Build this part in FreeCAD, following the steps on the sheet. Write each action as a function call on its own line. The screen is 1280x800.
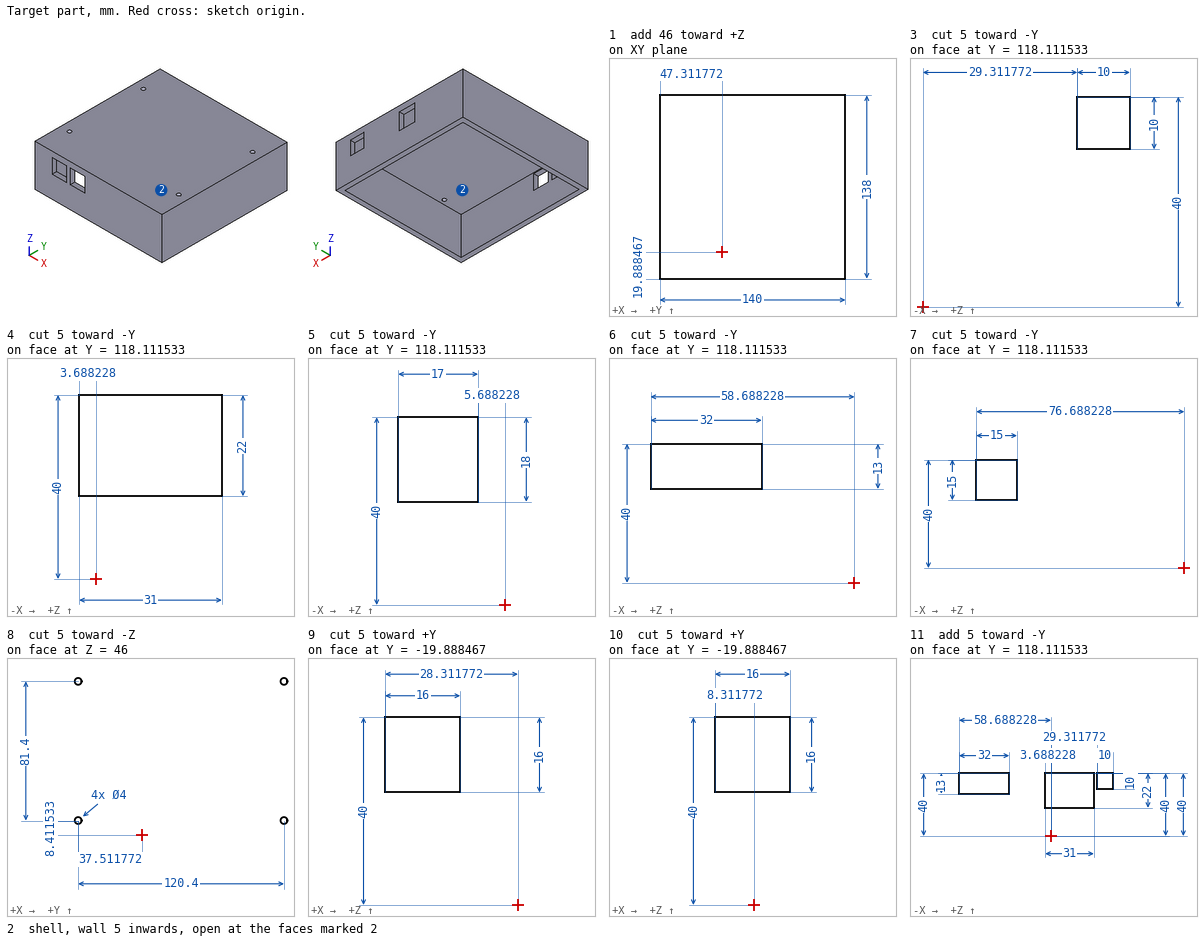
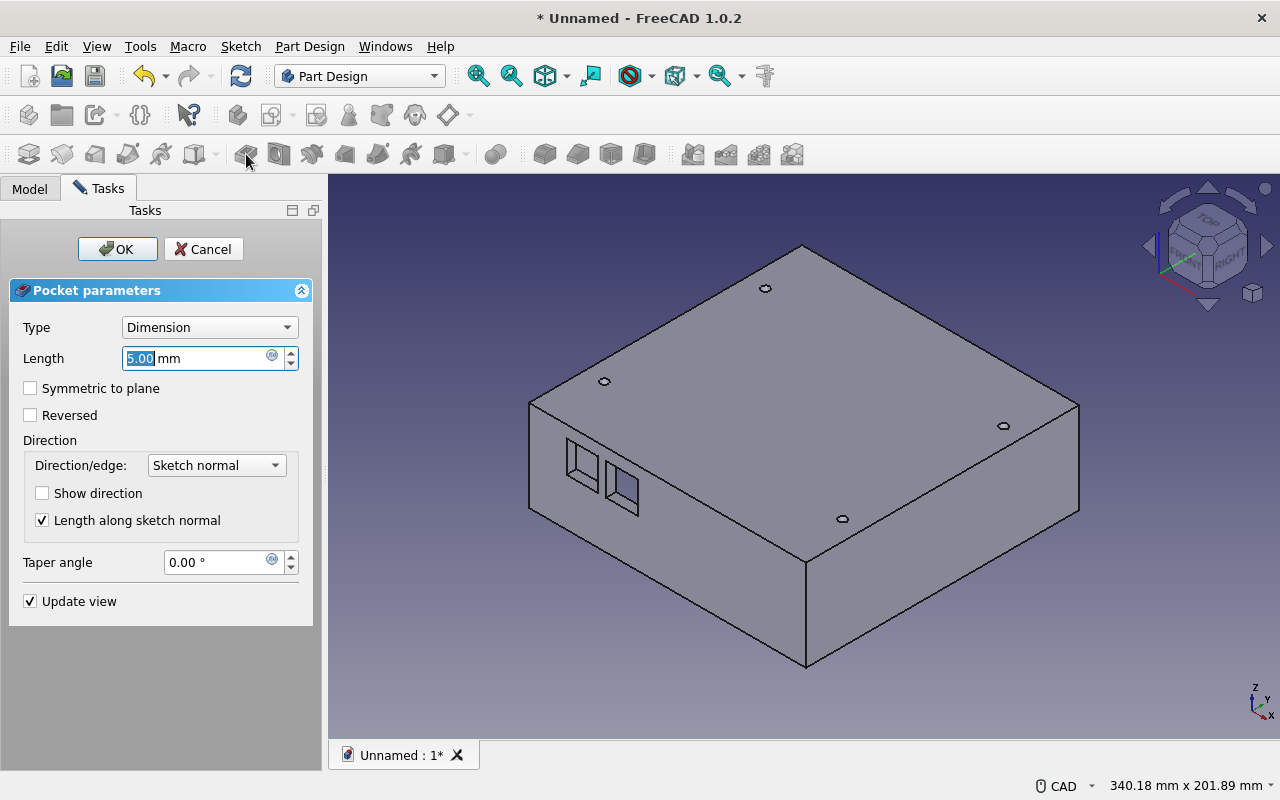
text(5)
key(Tab)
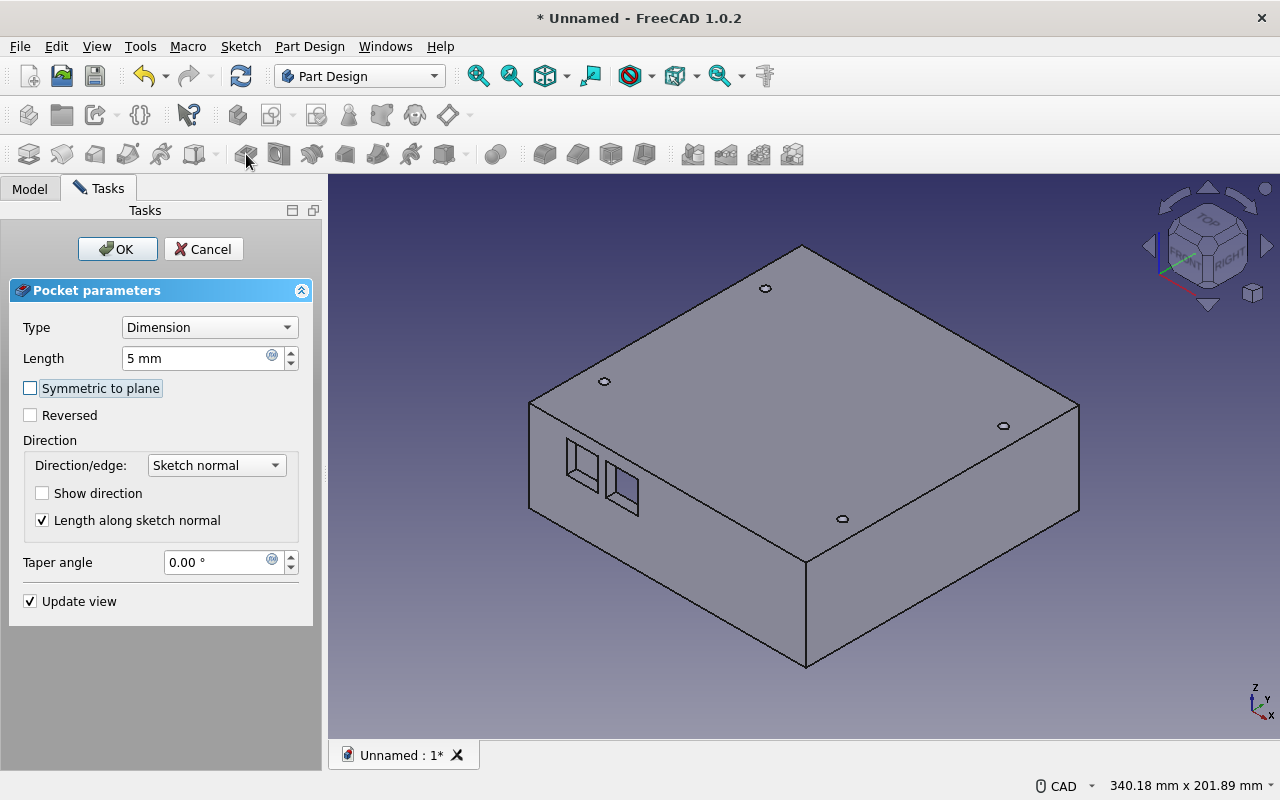
click(118, 249)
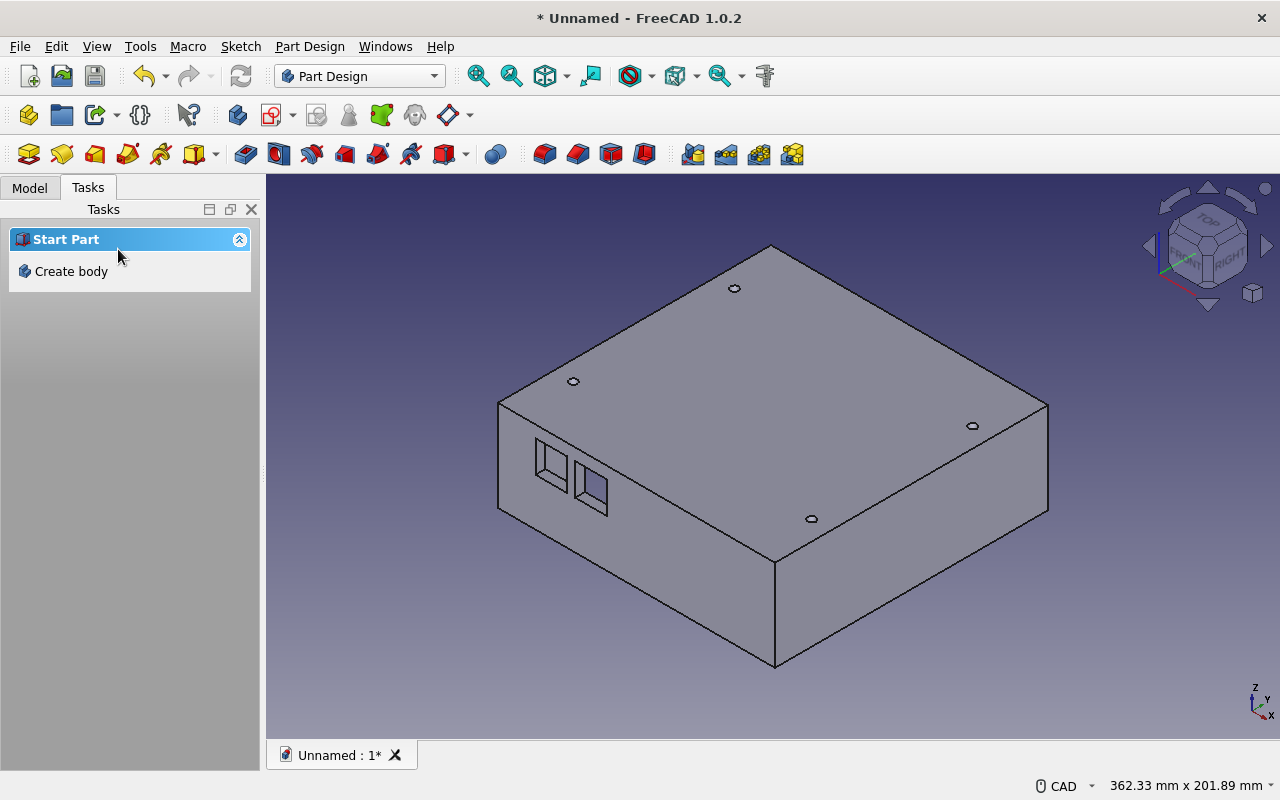
key(4)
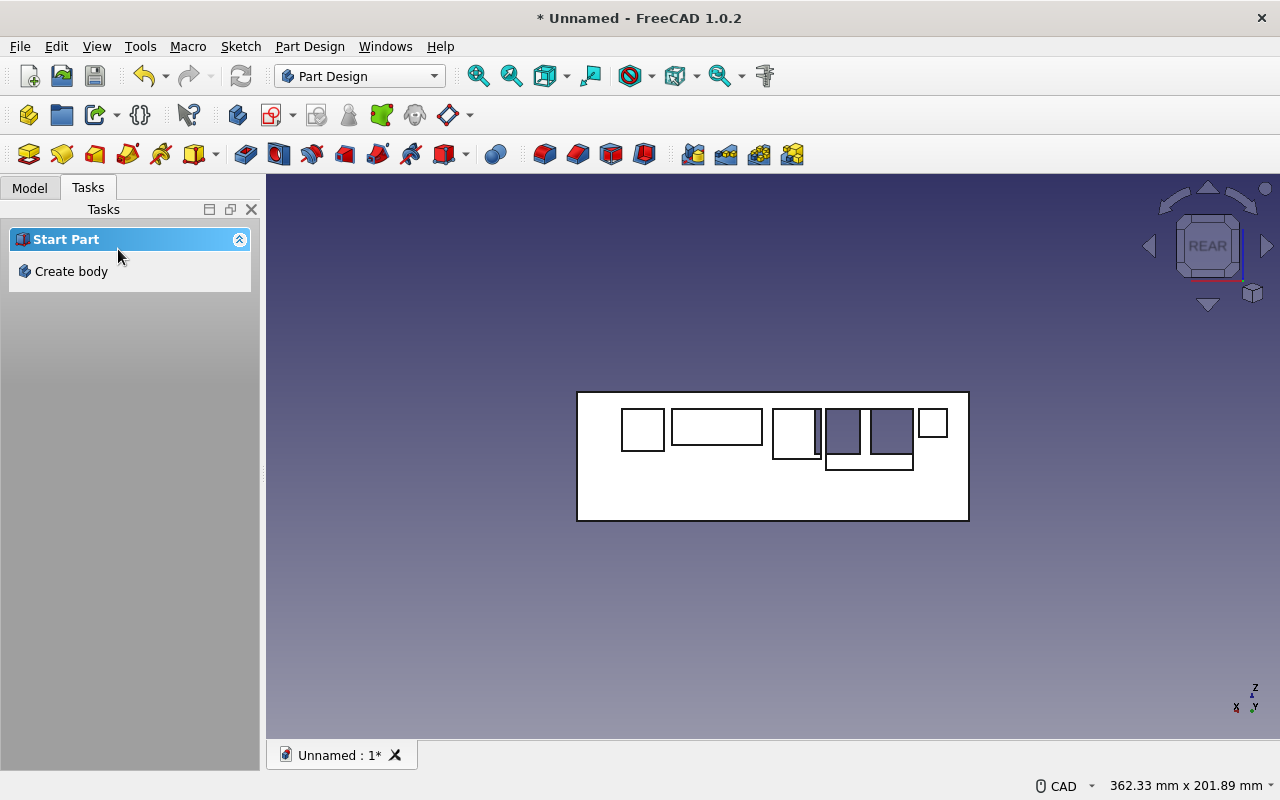
key(v)
key(f)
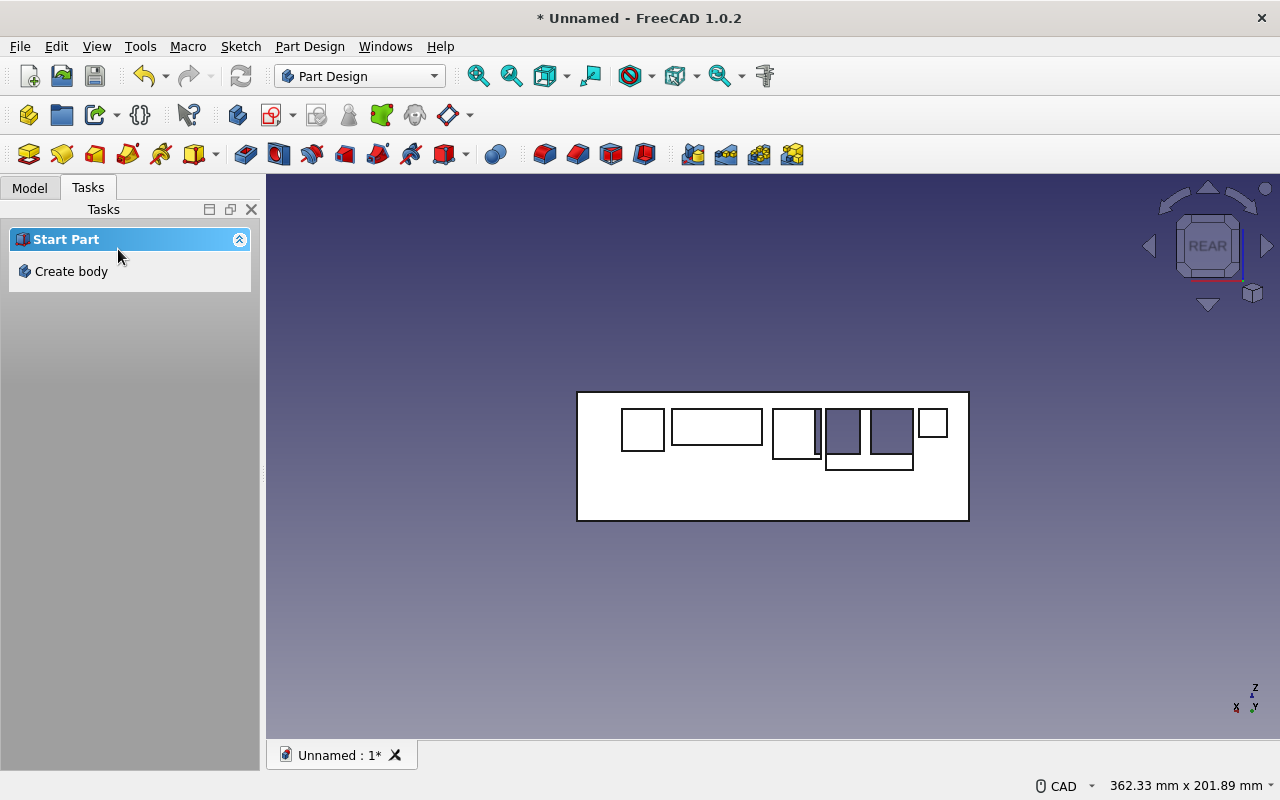
click(717, 474)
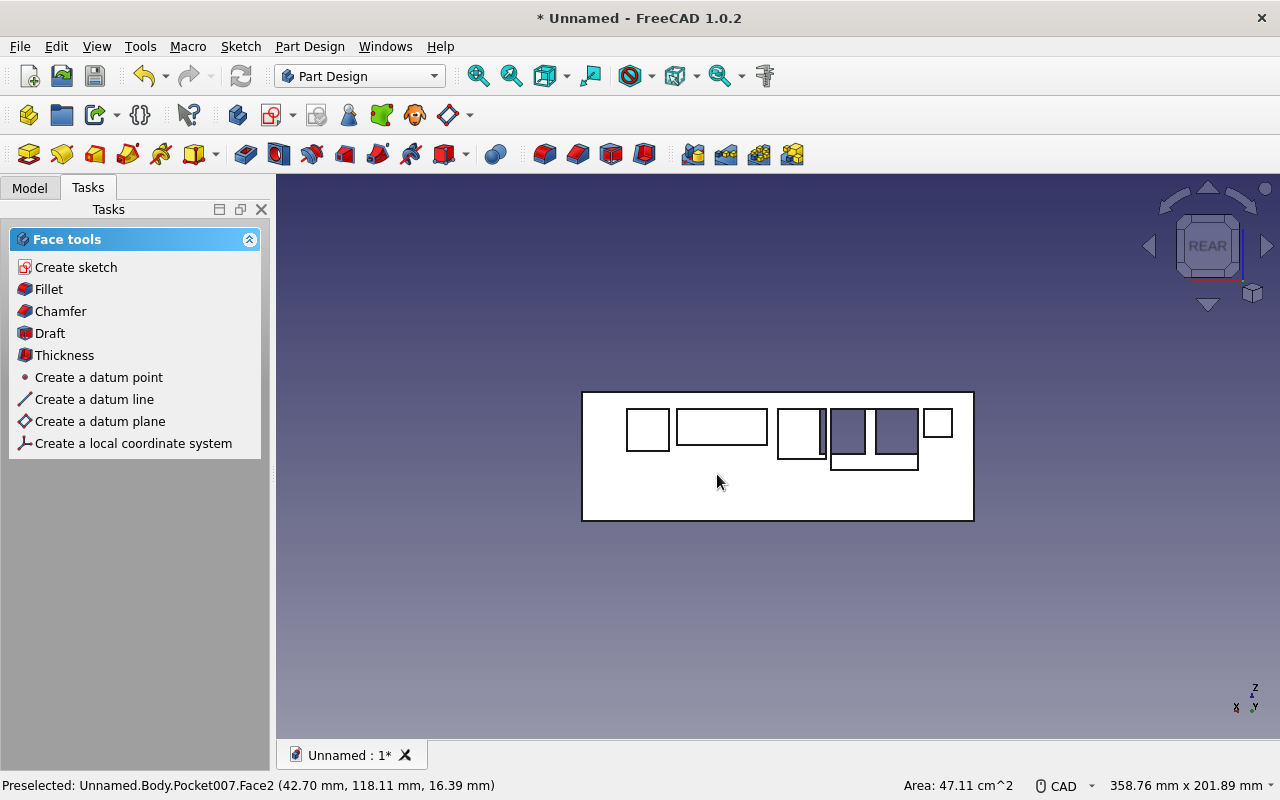
click(270, 116)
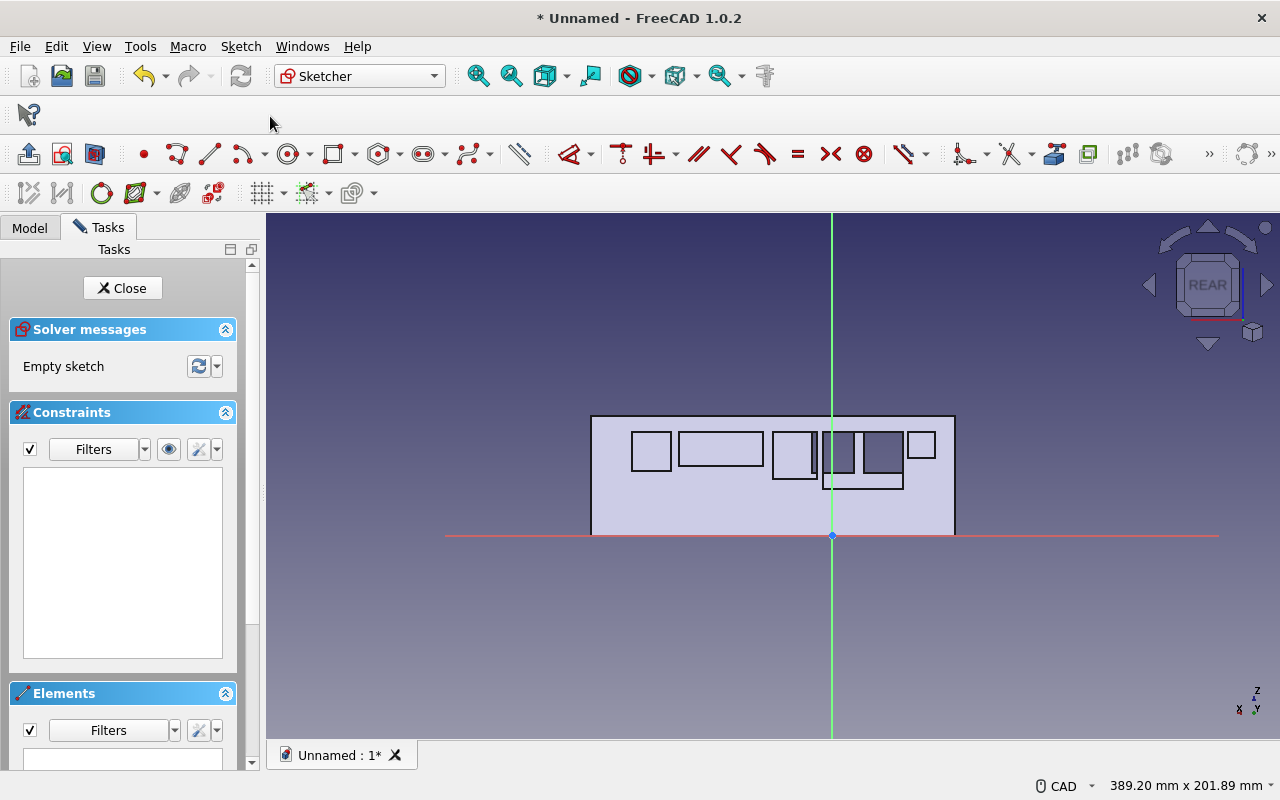
scroll(890, 490, up, 4)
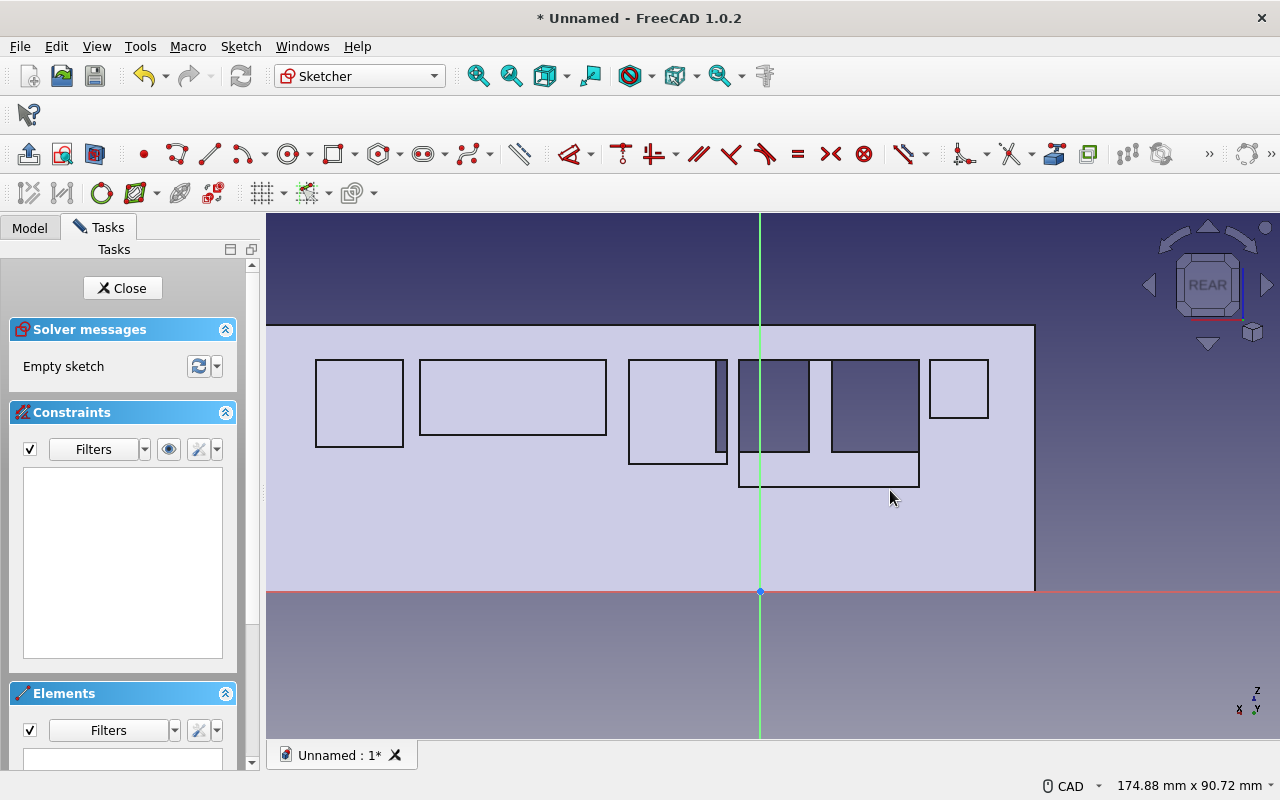
key(g)
key(r)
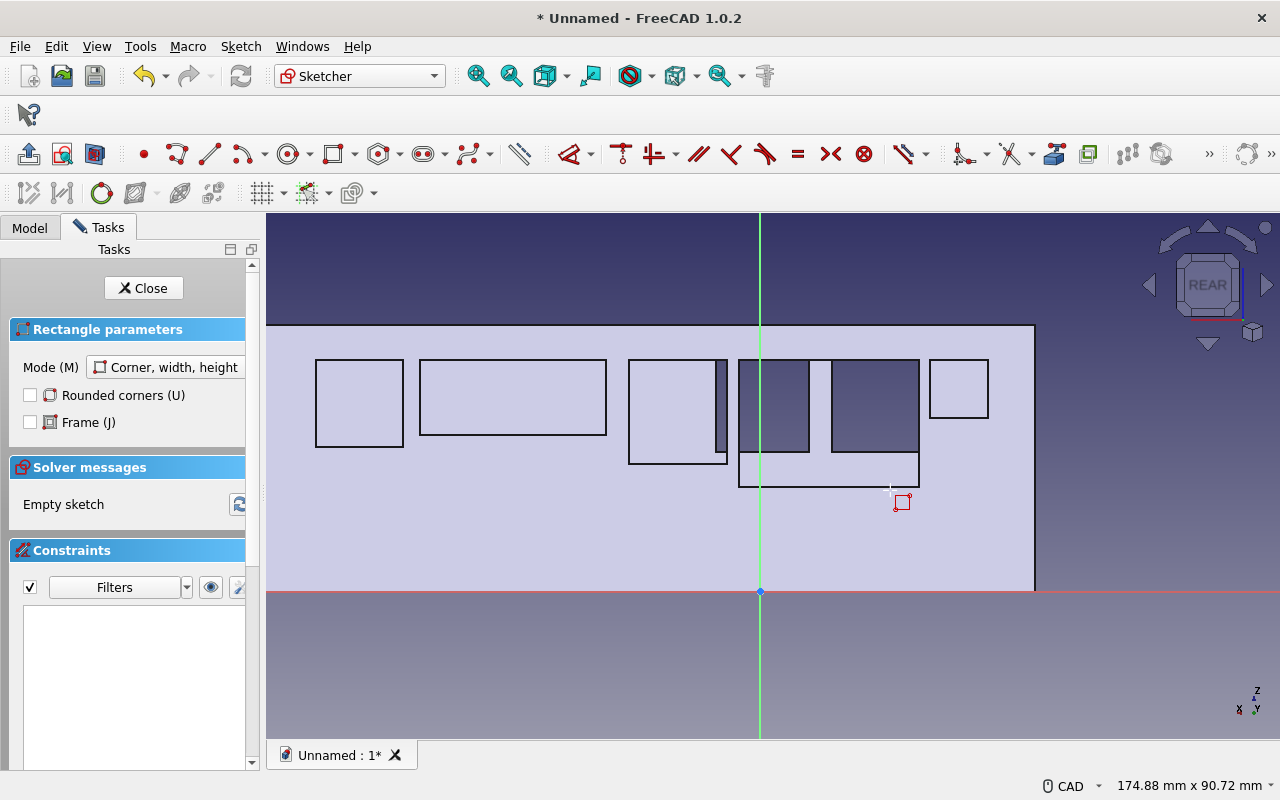
click(930, 360)
move(988, 418)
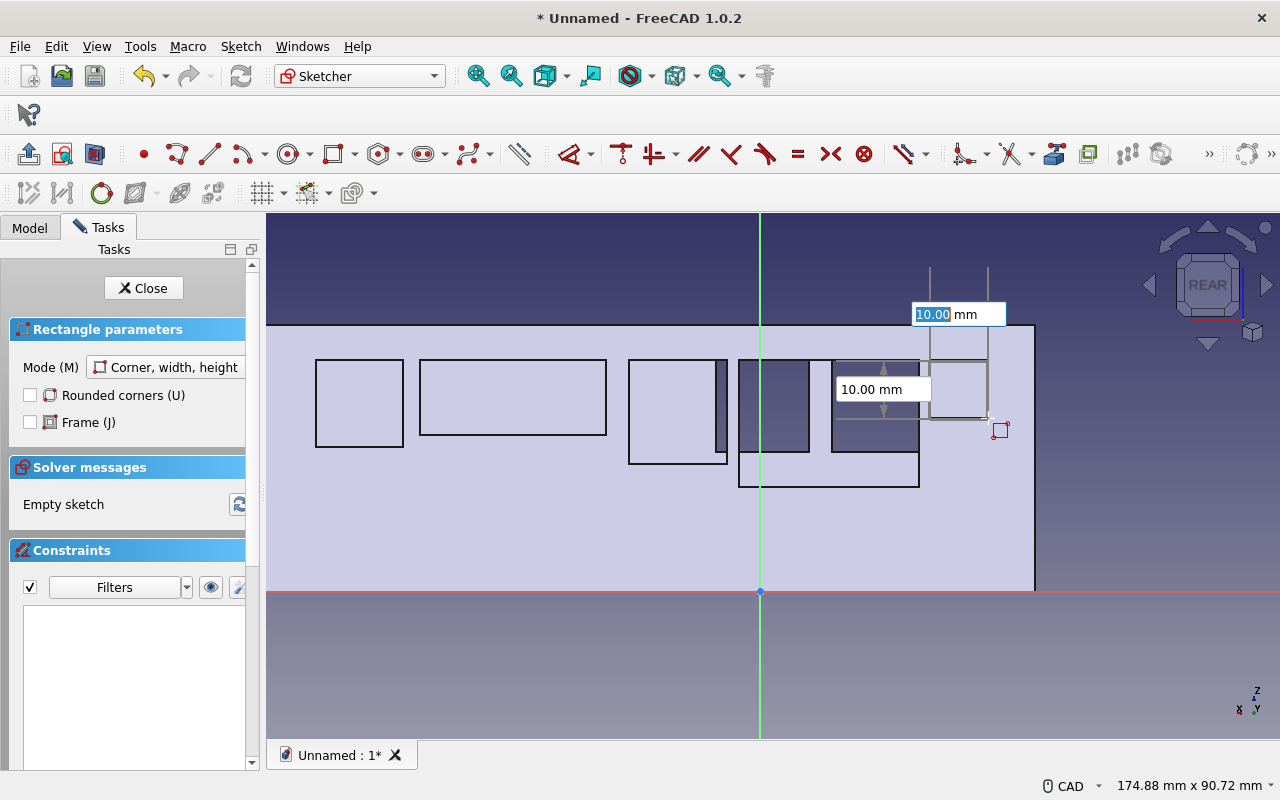
text(10)
key(Tab)
text(10)
key(Return)